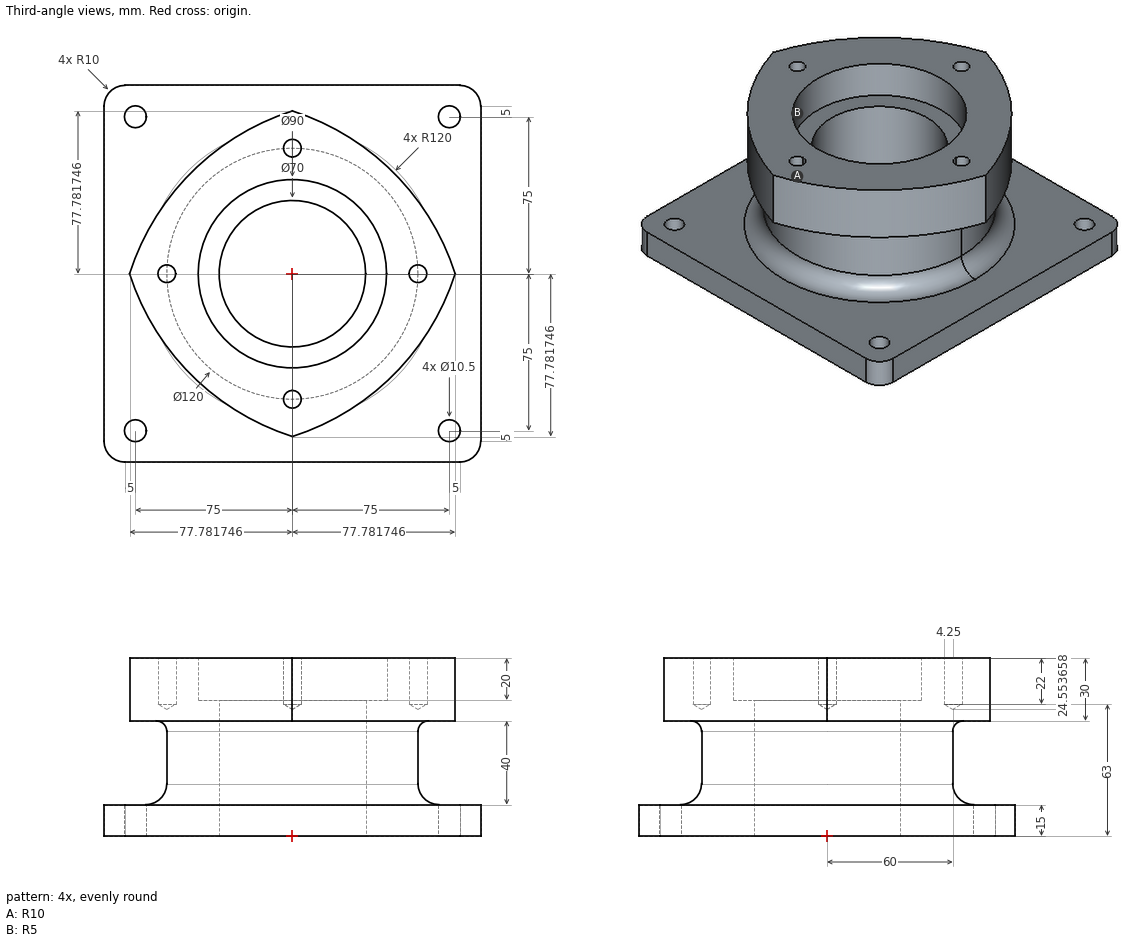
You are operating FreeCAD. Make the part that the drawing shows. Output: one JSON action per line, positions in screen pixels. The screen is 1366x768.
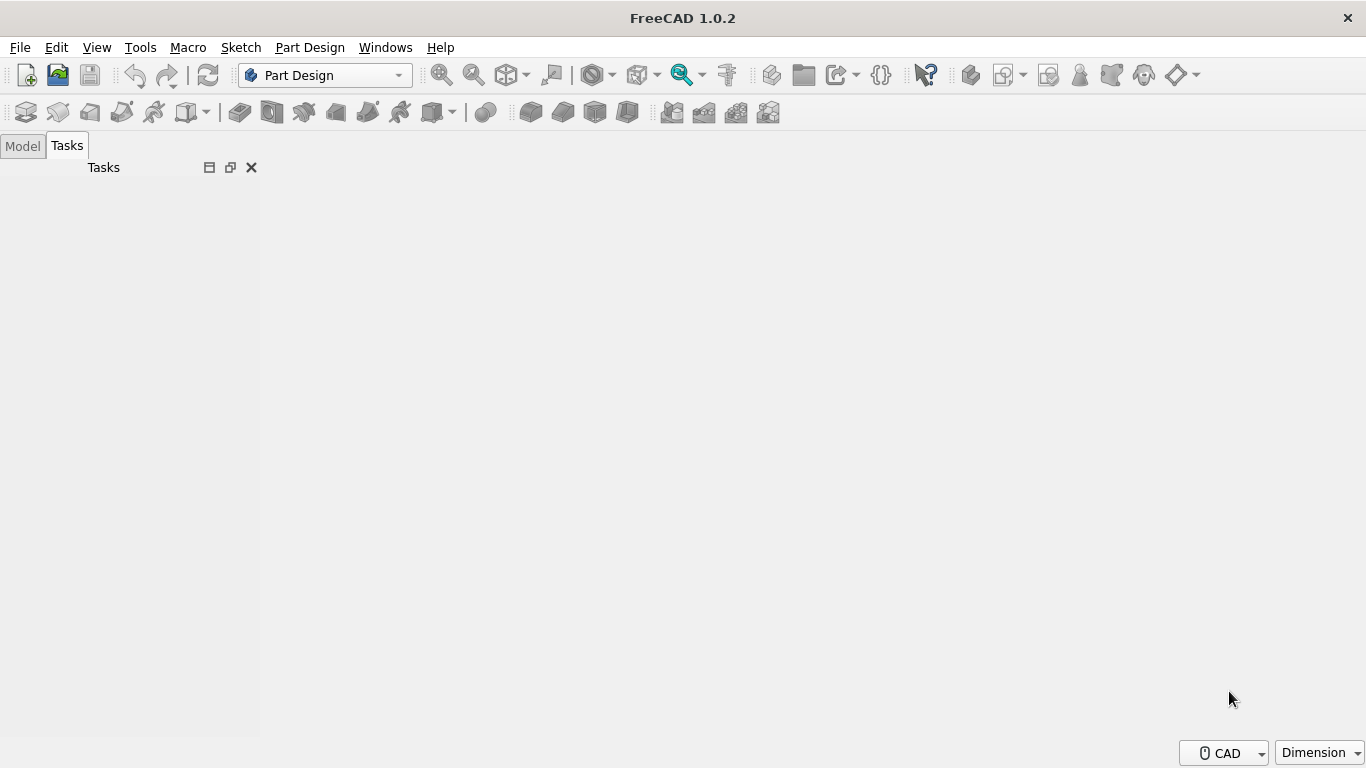
{"action": "left_click", "coordinate": [26, 76]}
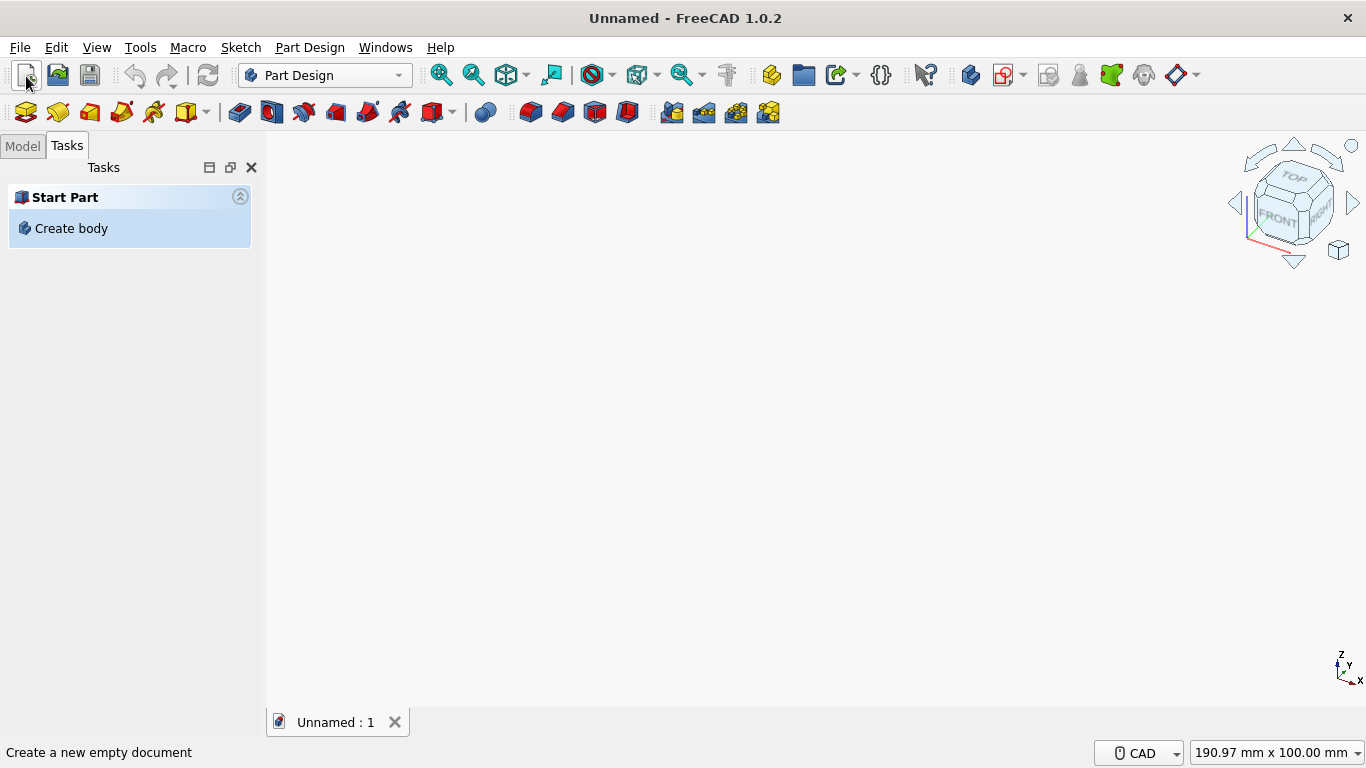
{"action": "left_click", "coordinate": [1004, 76]}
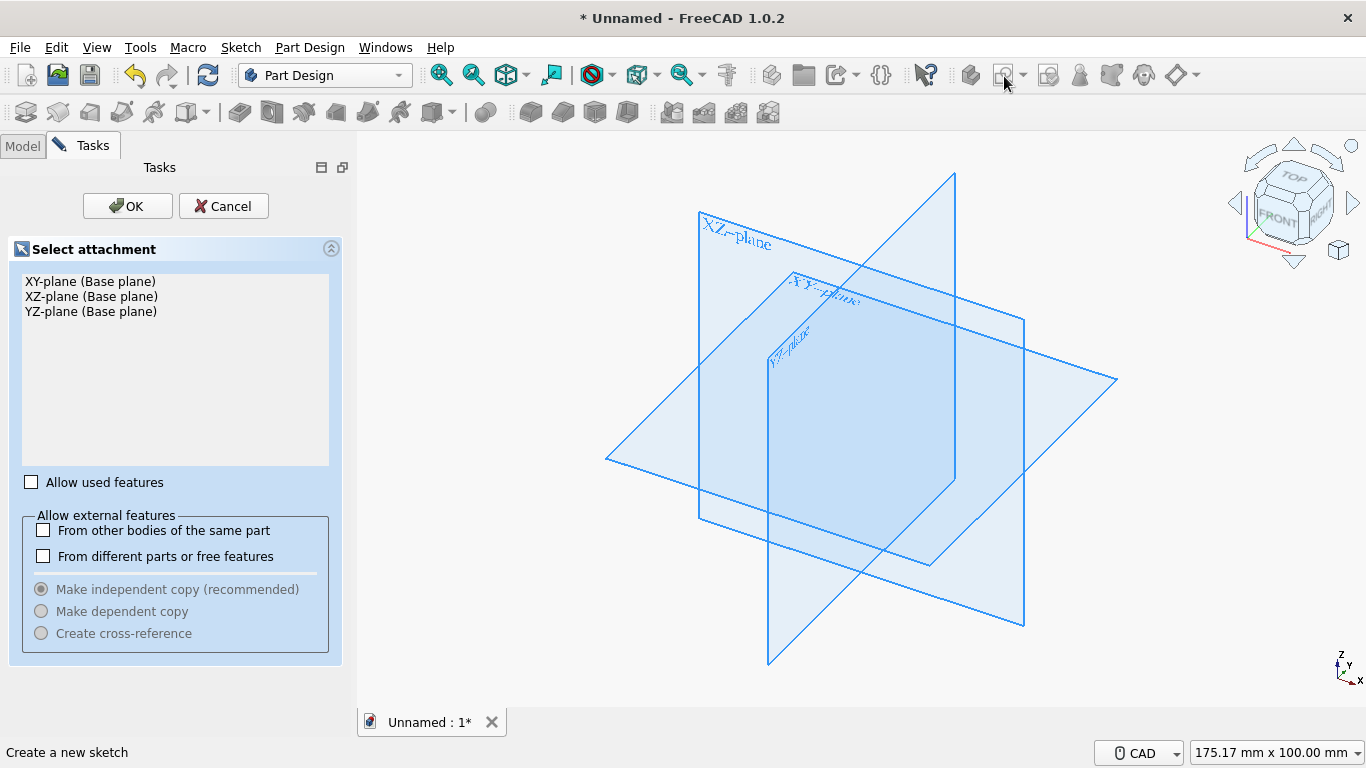
{"action": "left_click", "coordinate": [82, 282]}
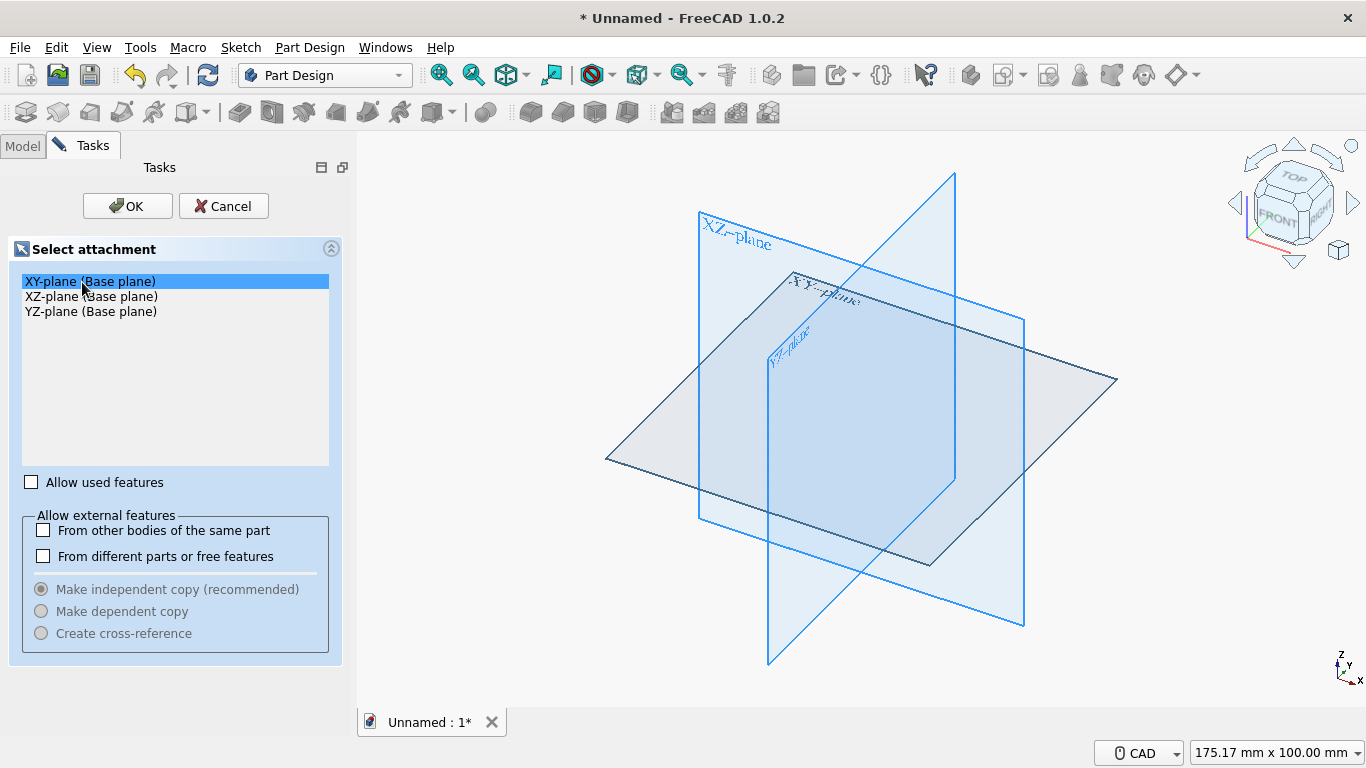
{"action": "left_click", "coordinate": [128, 206]}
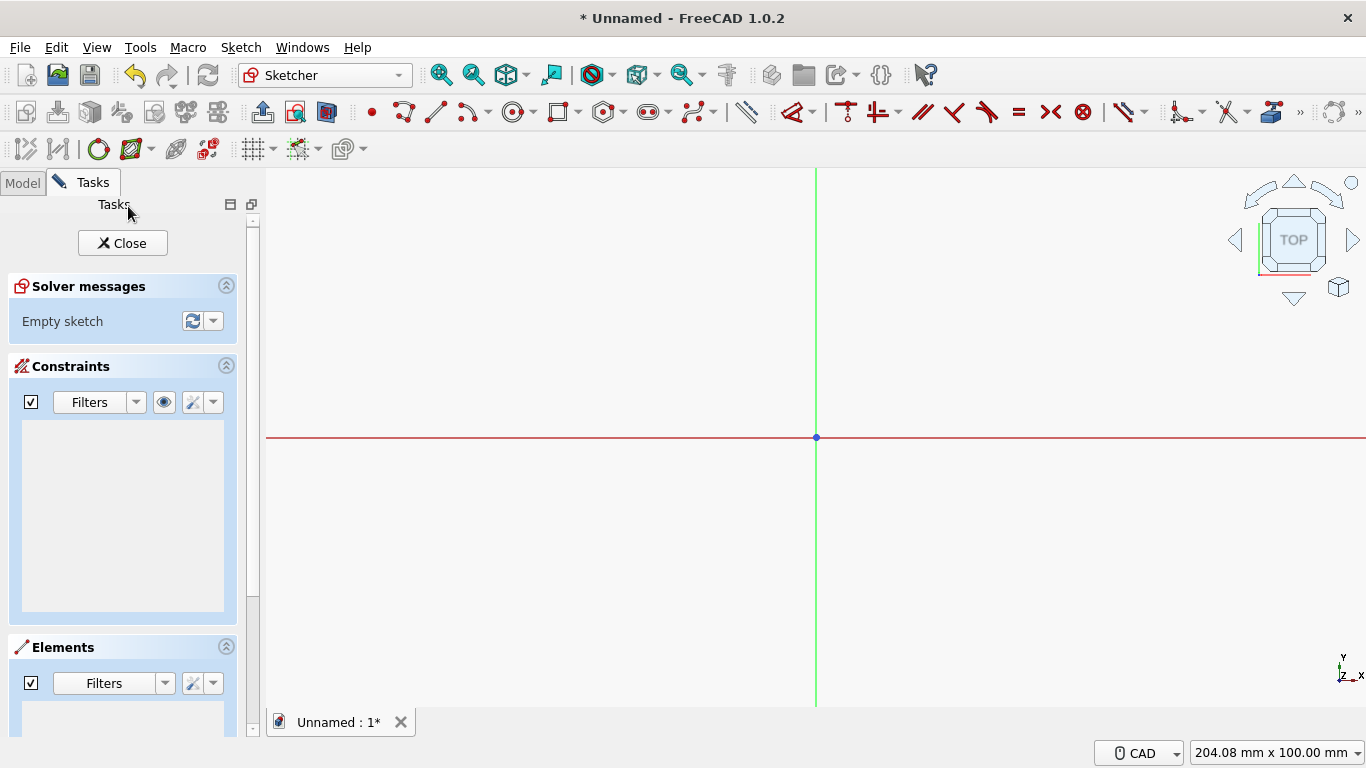
{"action": "scroll", "coordinate": [708, 438], "scroll_direction": "down", "scroll_amount": 5}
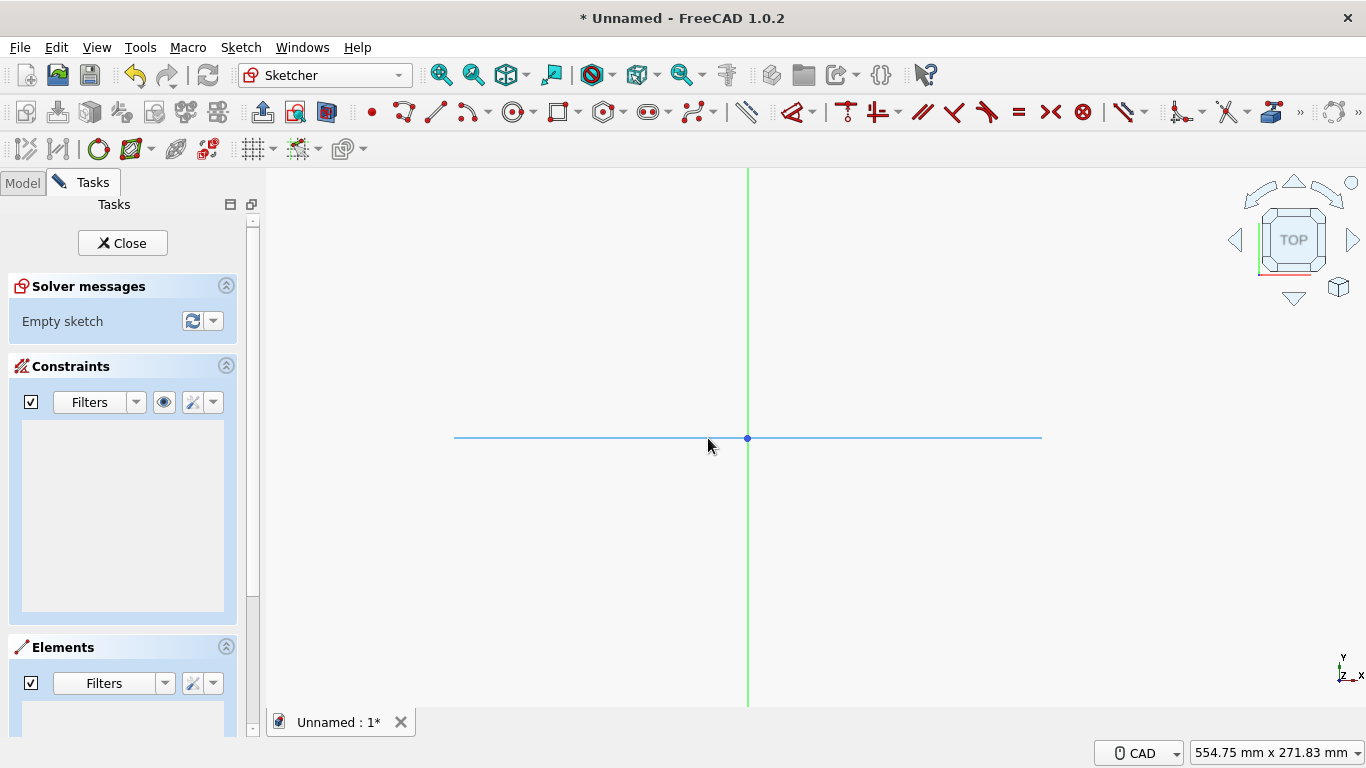
{"action": "left_click", "coordinate": [436, 112]}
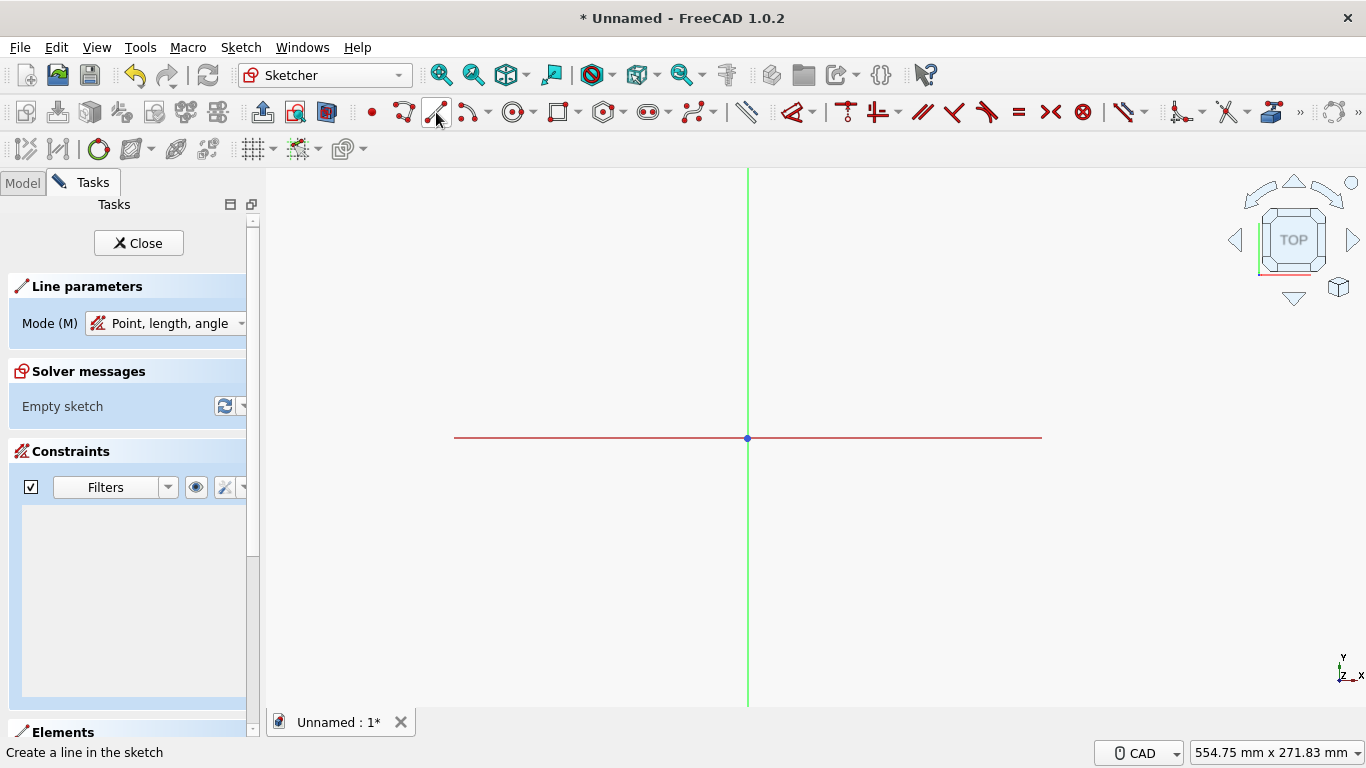
{"action": "left_click", "coordinate": [907, 260]}
{"action": "left_click", "coordinate": [589, 260]}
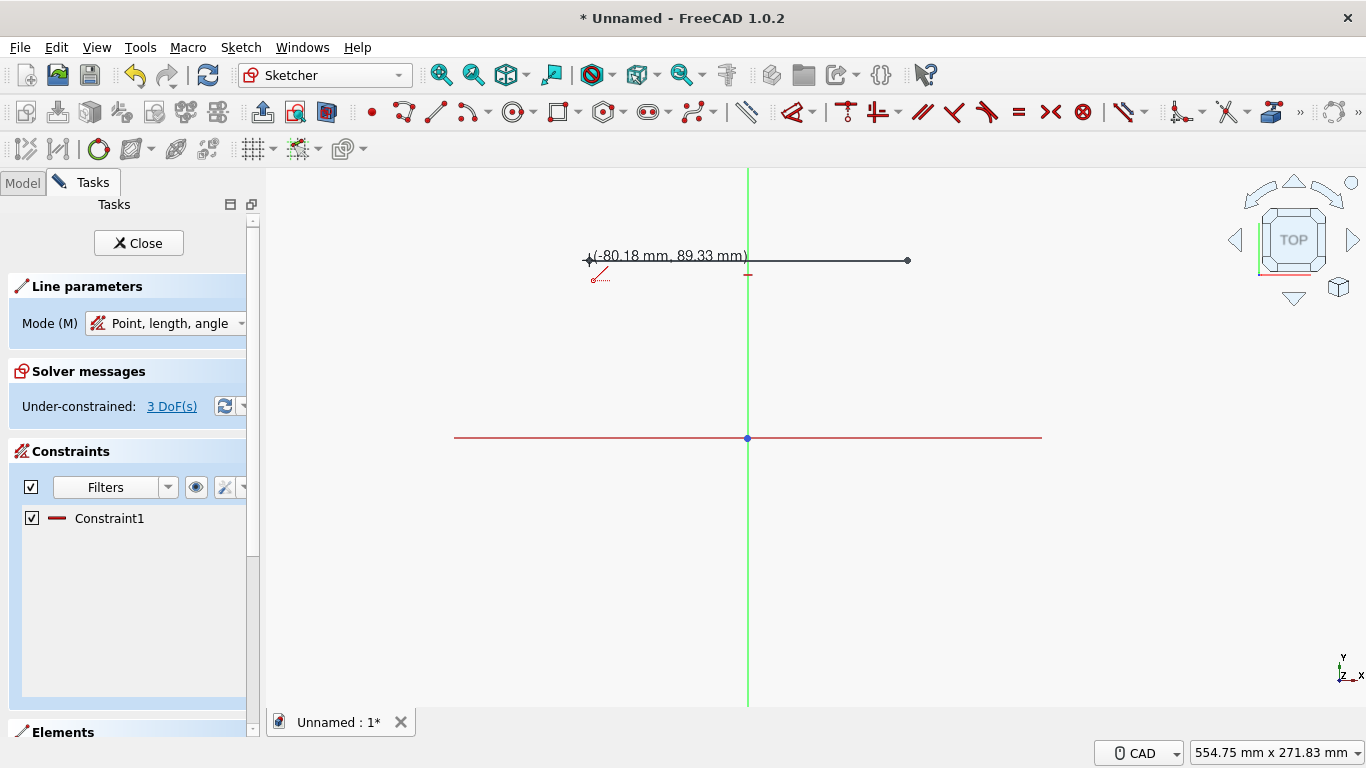
{"action": "left_click", "coordinate": [570, 280]}
{"action": "left_click", "coordinate": [570, 597]}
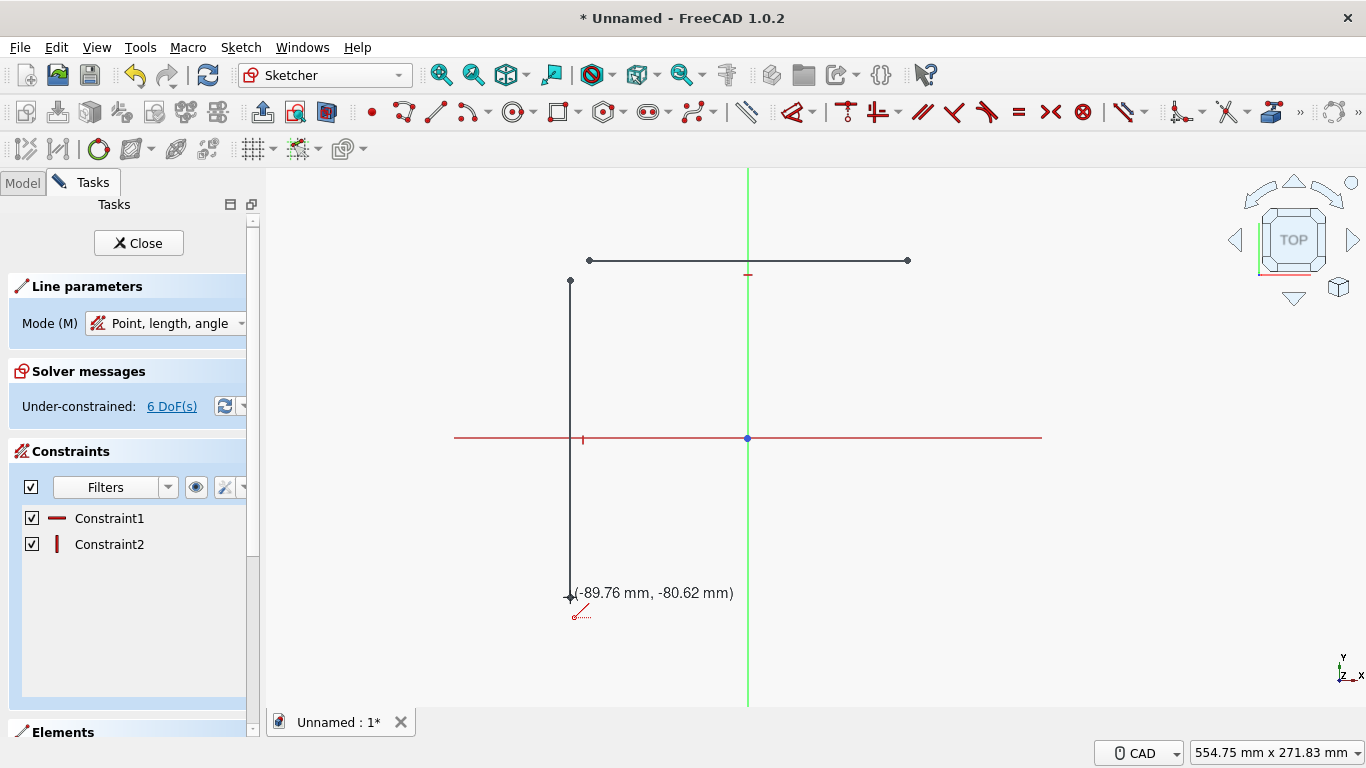
{"action": "left_click", "coordinate": [589, 617]}
{"action": "left_click", "coordinate": [907, 617]}